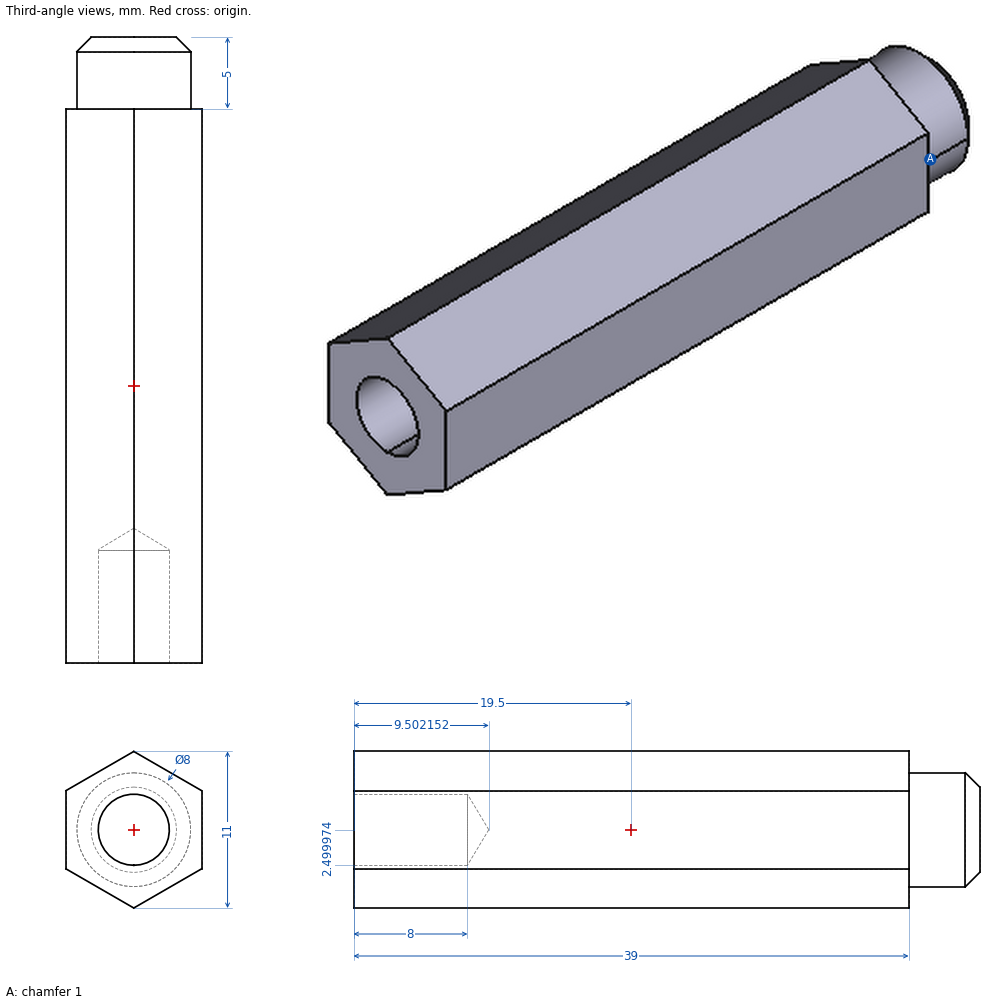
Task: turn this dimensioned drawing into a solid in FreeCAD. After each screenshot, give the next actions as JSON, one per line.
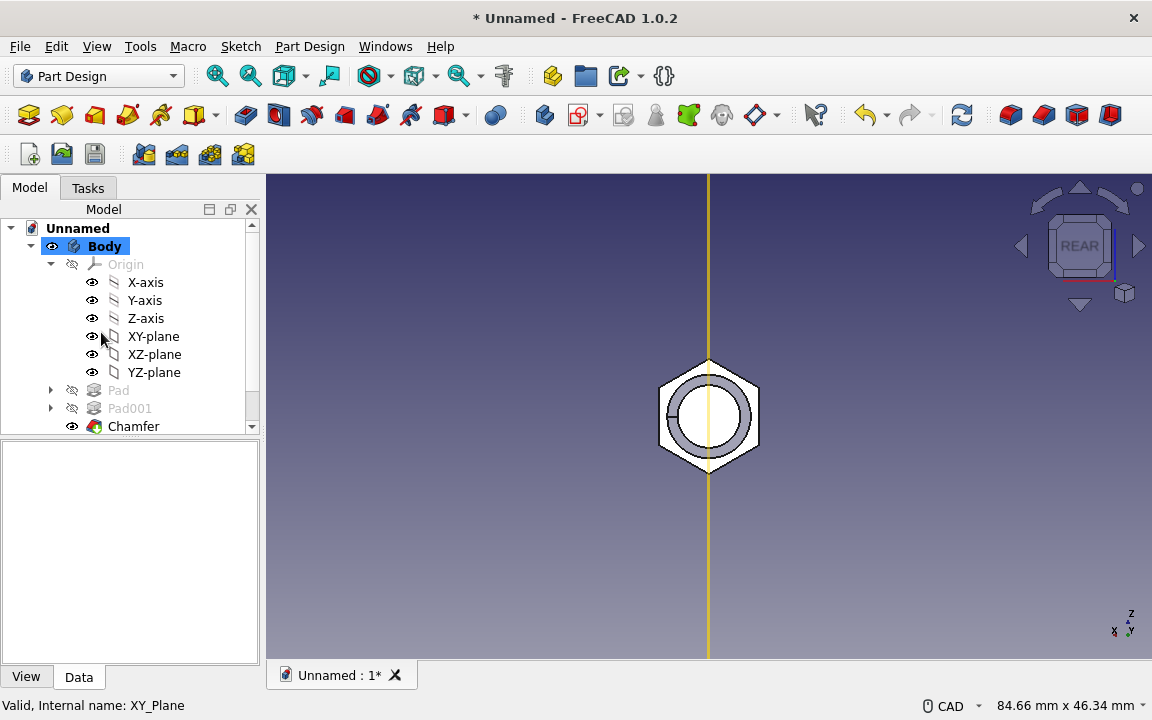
{"action": "left_click", "coordinate": [117, 408]}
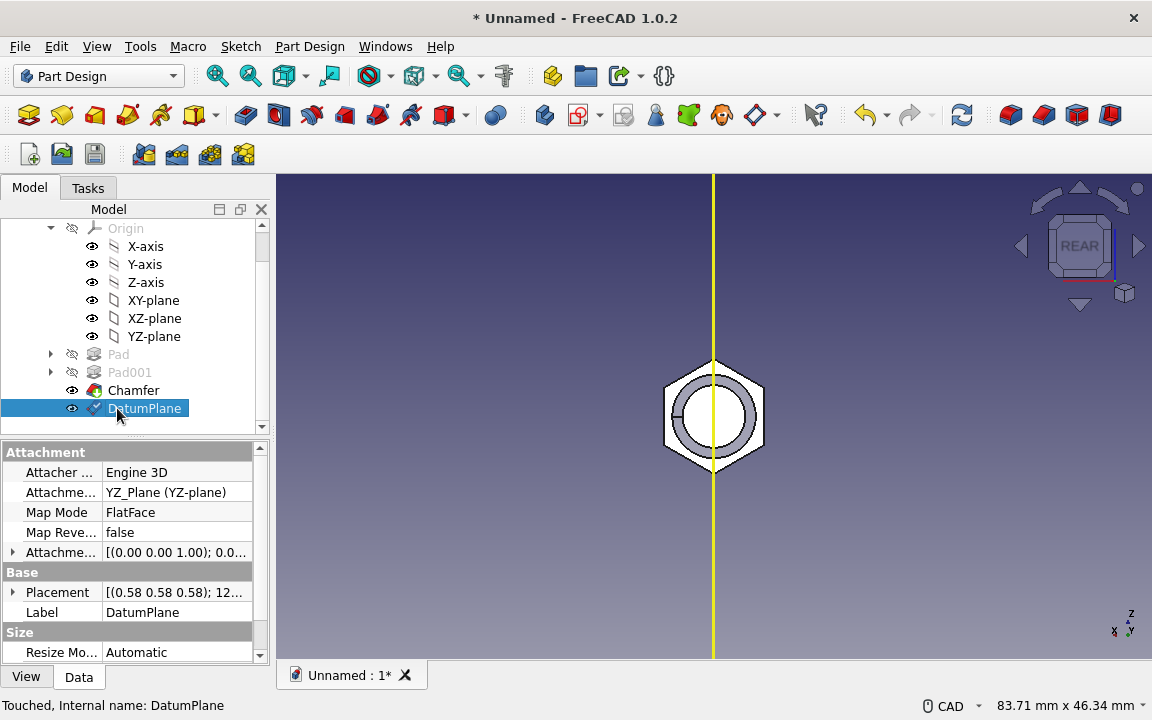
{"action": "left_click", "coordinate": [578, 116]}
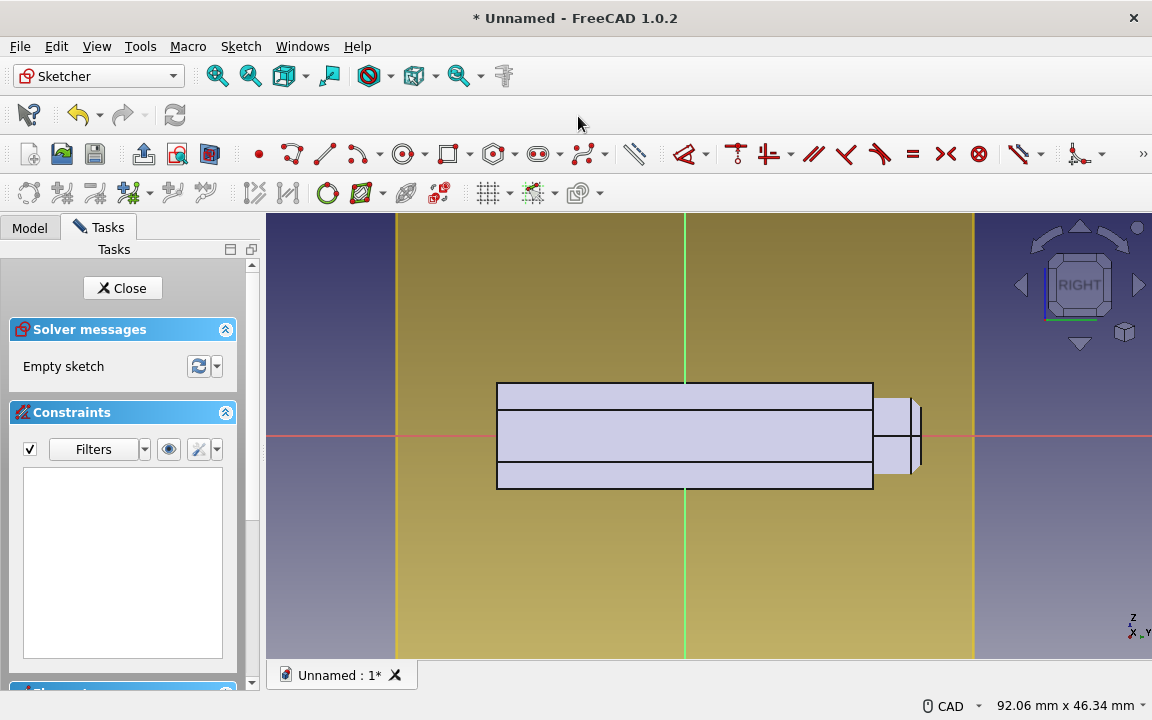
{"action": "key", "text": "q s"}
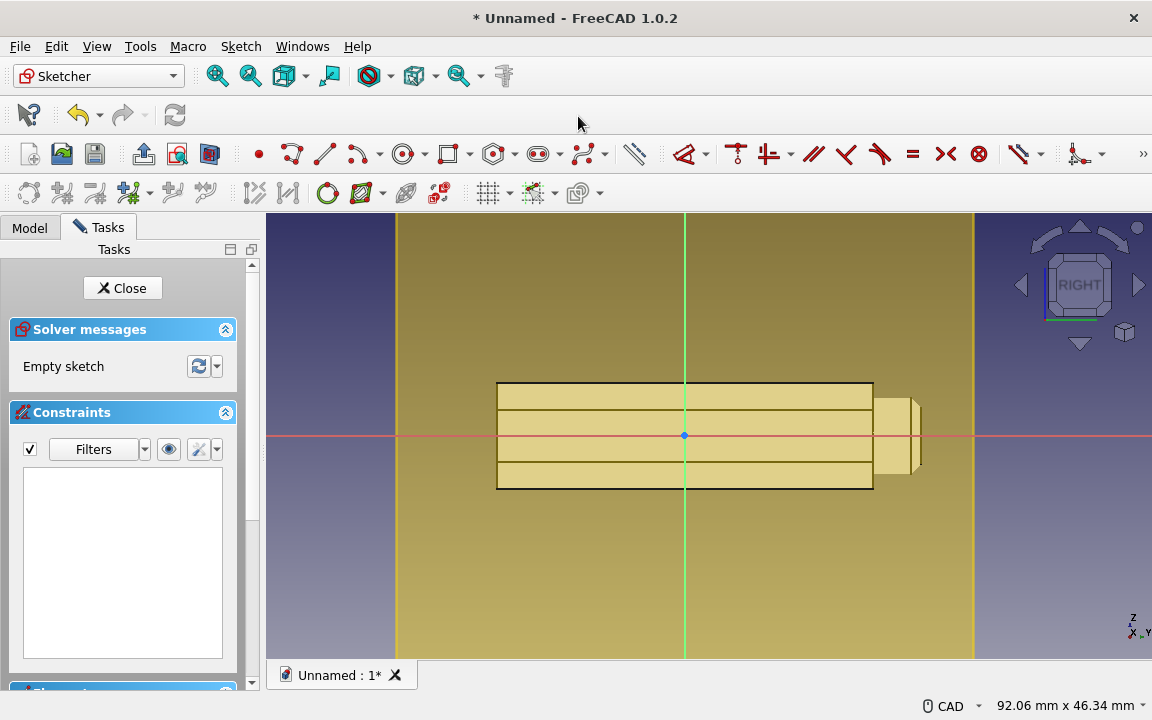
{"action": "scroll", "coordinate": [555, 455], "scroll_direction": "up", "scroll_amount": 5}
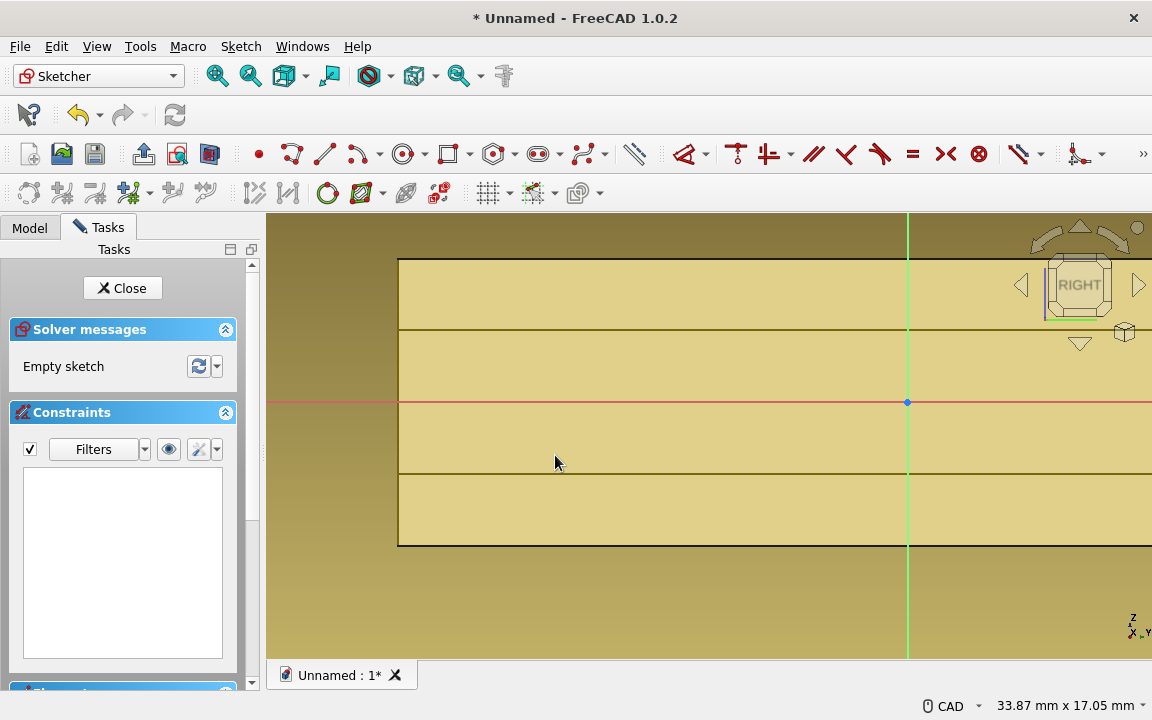
{"action": "left_click", "coordinate": [292, 154]}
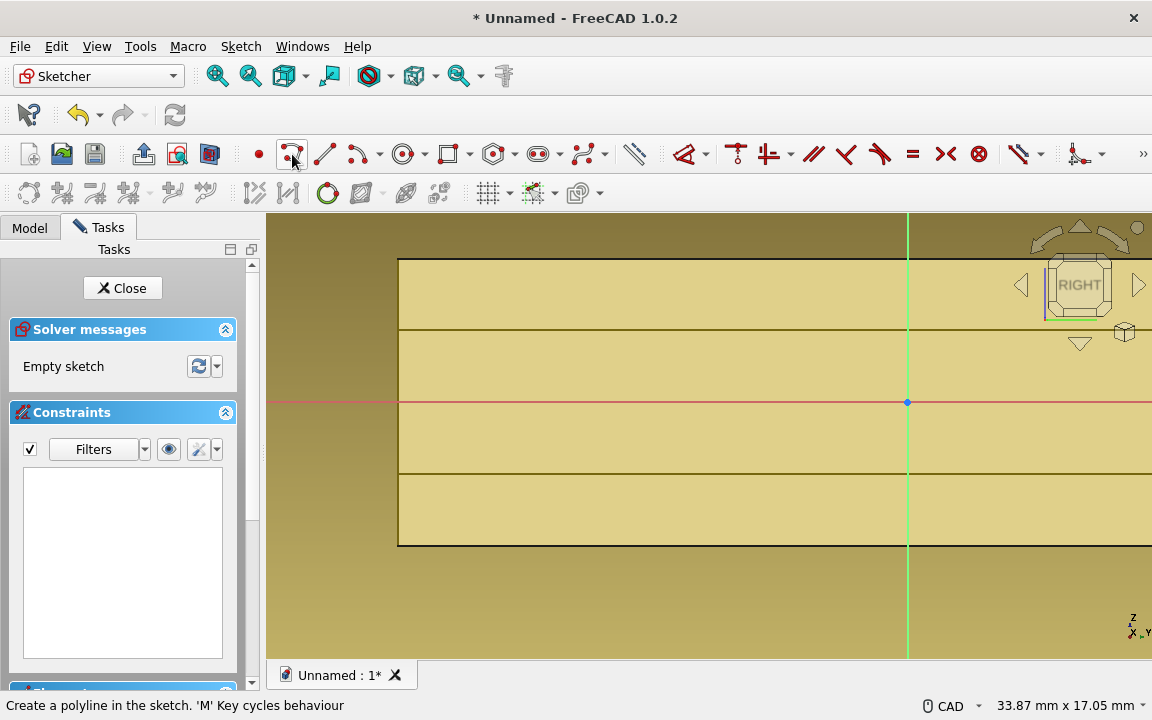
{"action": "left_click", "coordinate": [646, 402]}
{"action": "left_click", "coordinate": [398, 411]}
{"action": "left_click", "coordinate": [398, 468]}
{"action": "left_click", "coordinate": [607, 468]}
{"action": "left_click", "coordinate": [646, 402]}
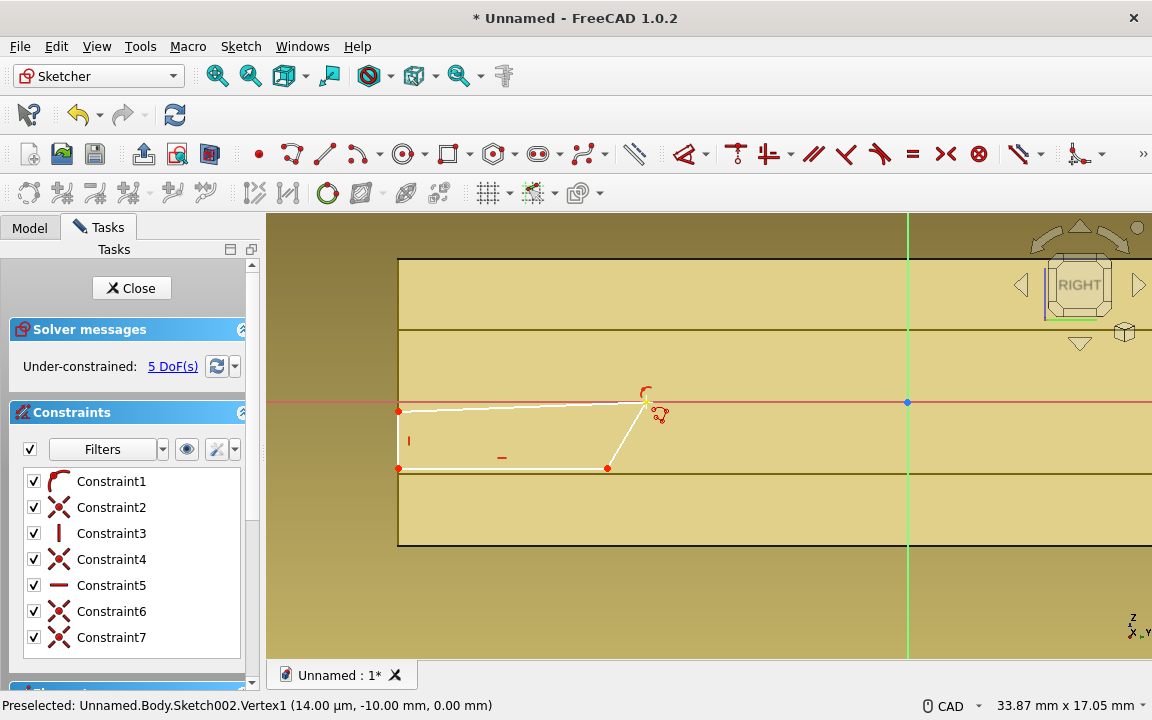
{"action": "key", "text": "g l"}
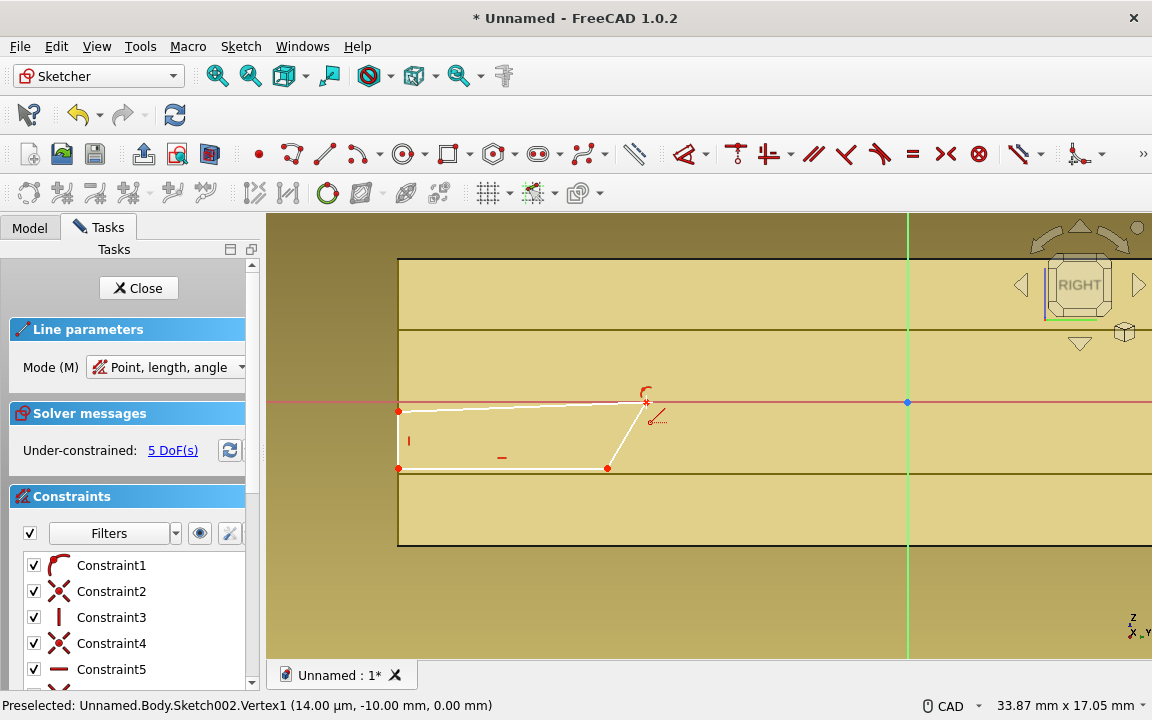
{"action": "left_click", "coordinate": [373, 402]}
{"action": "left_click", "coordinate": [671, 402]}
{"action": "key", "text": "Escape"}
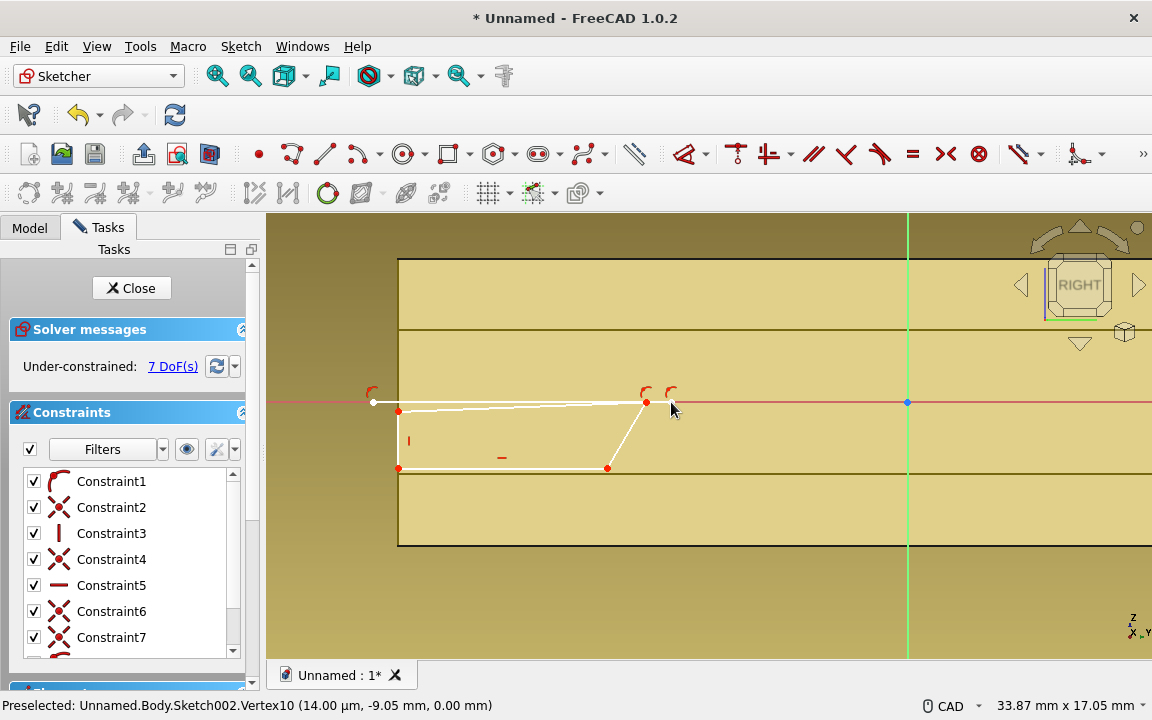
{"action": "scroll", "coordinate": [433, 402], "scroll_direction": "up", "scroll_amount": 3}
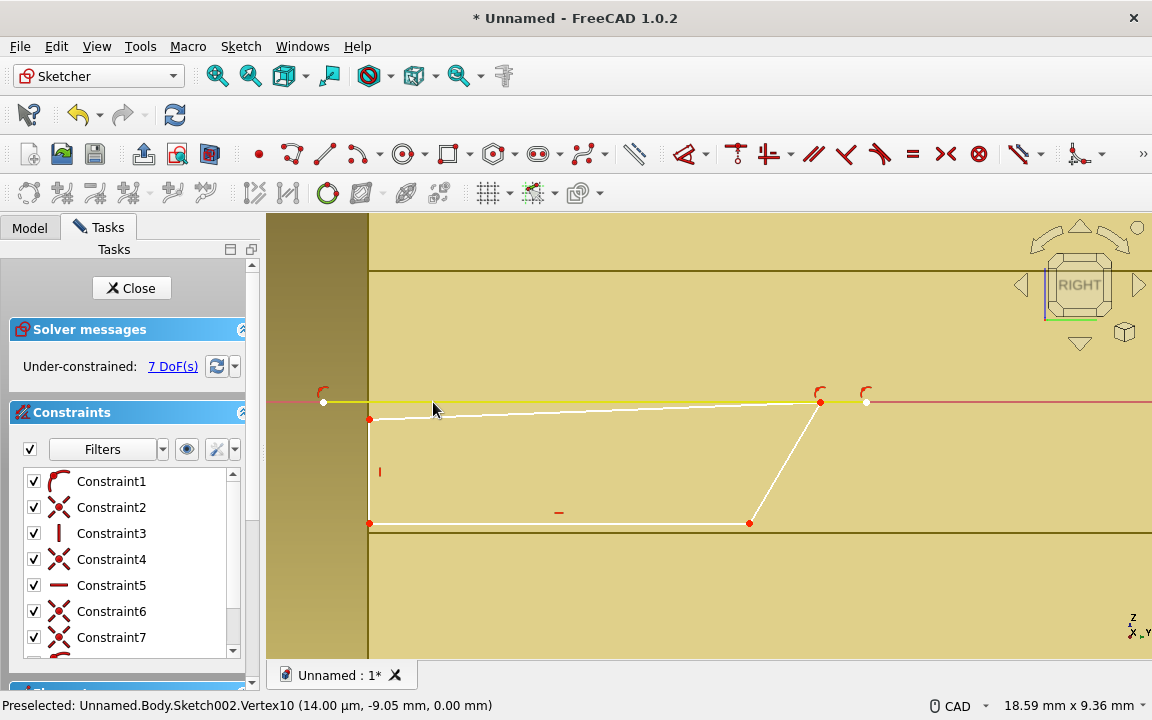
{"action": "left_click", "coordinate": [432, 402]}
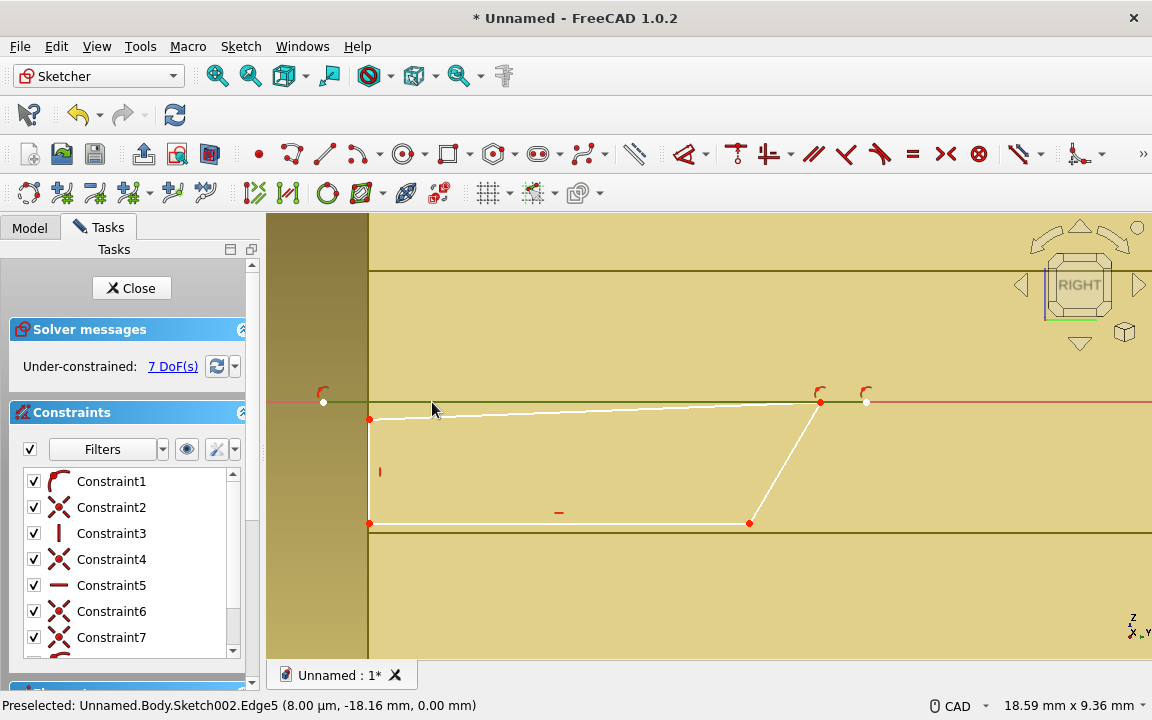
{"action": "left_click", "coordinate": [635, 154]}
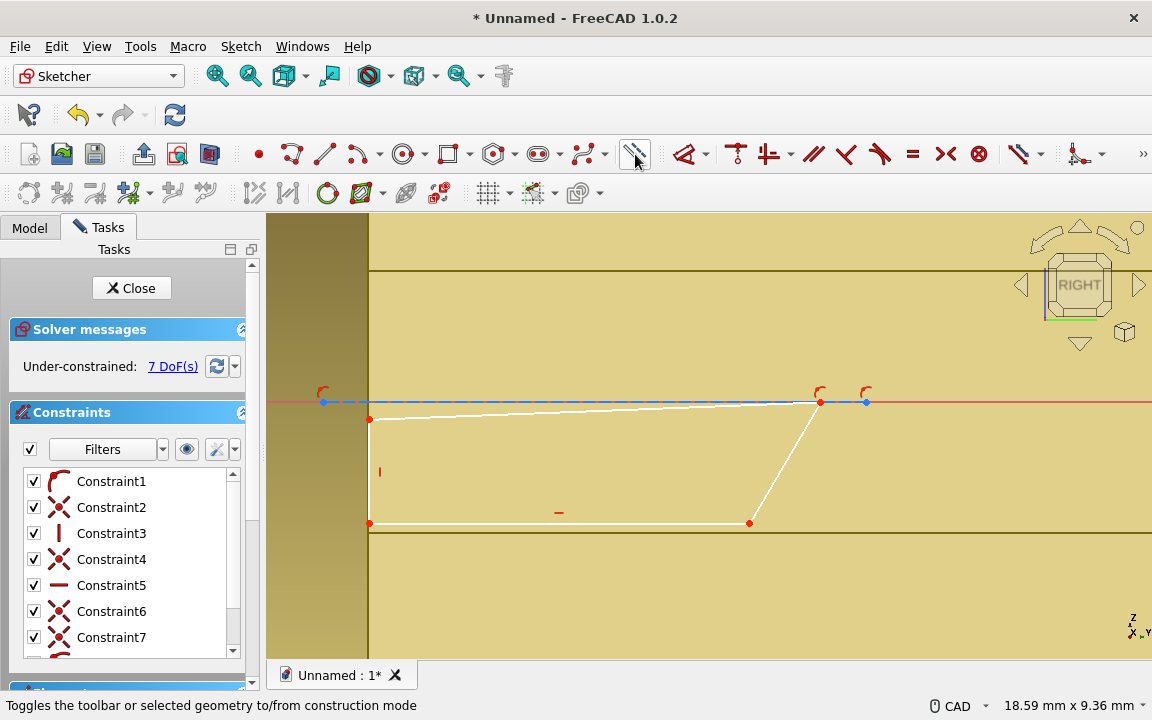
{"action": "left_click", "coordinate": [505, 415]}